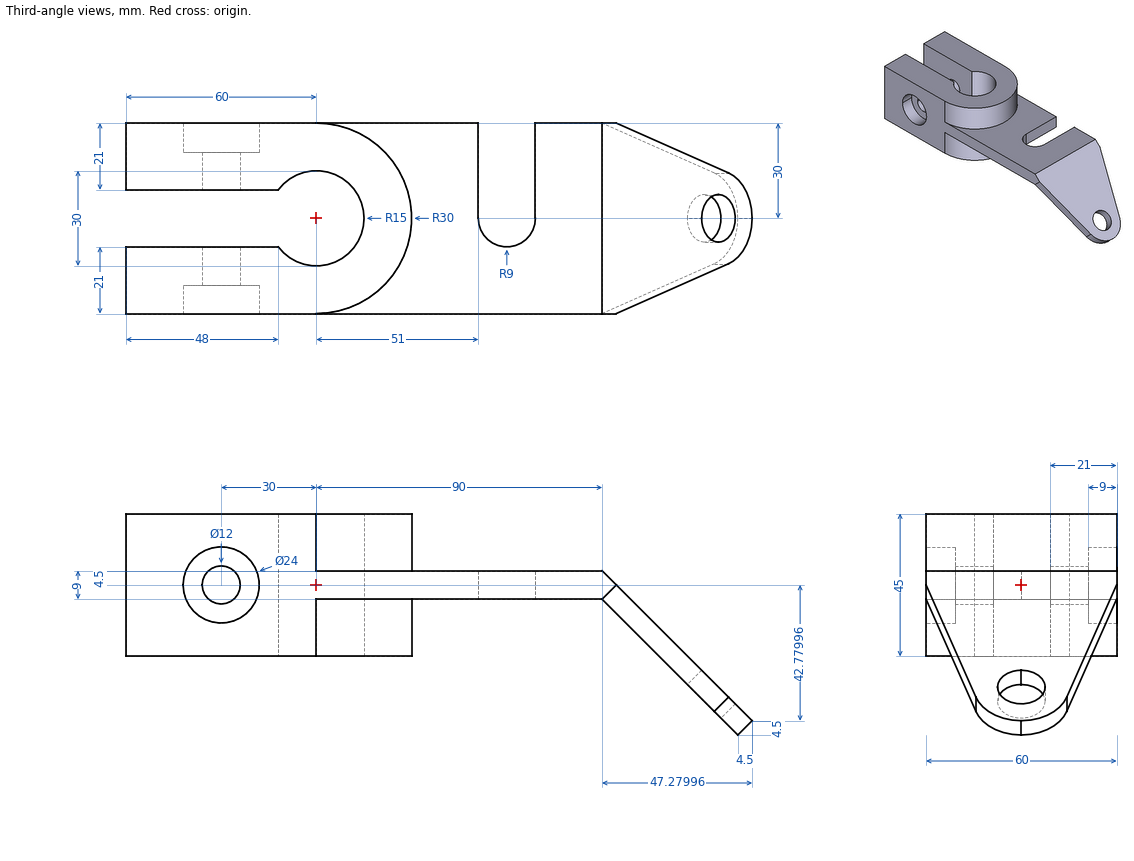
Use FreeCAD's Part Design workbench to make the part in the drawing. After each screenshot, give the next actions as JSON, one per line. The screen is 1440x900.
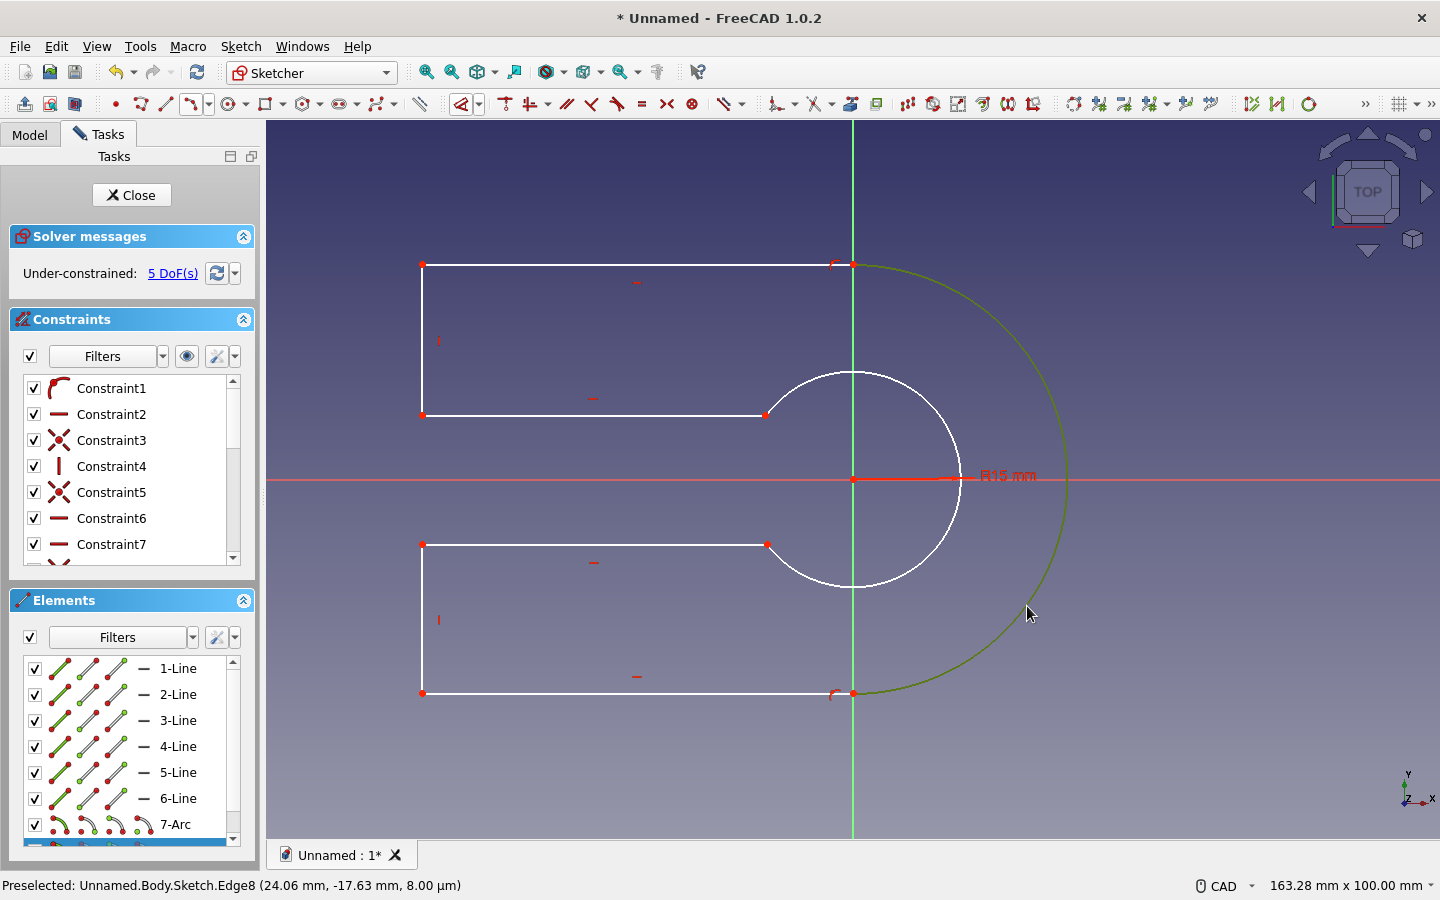
{"action": "left_click", "coordinate": [478, 104]}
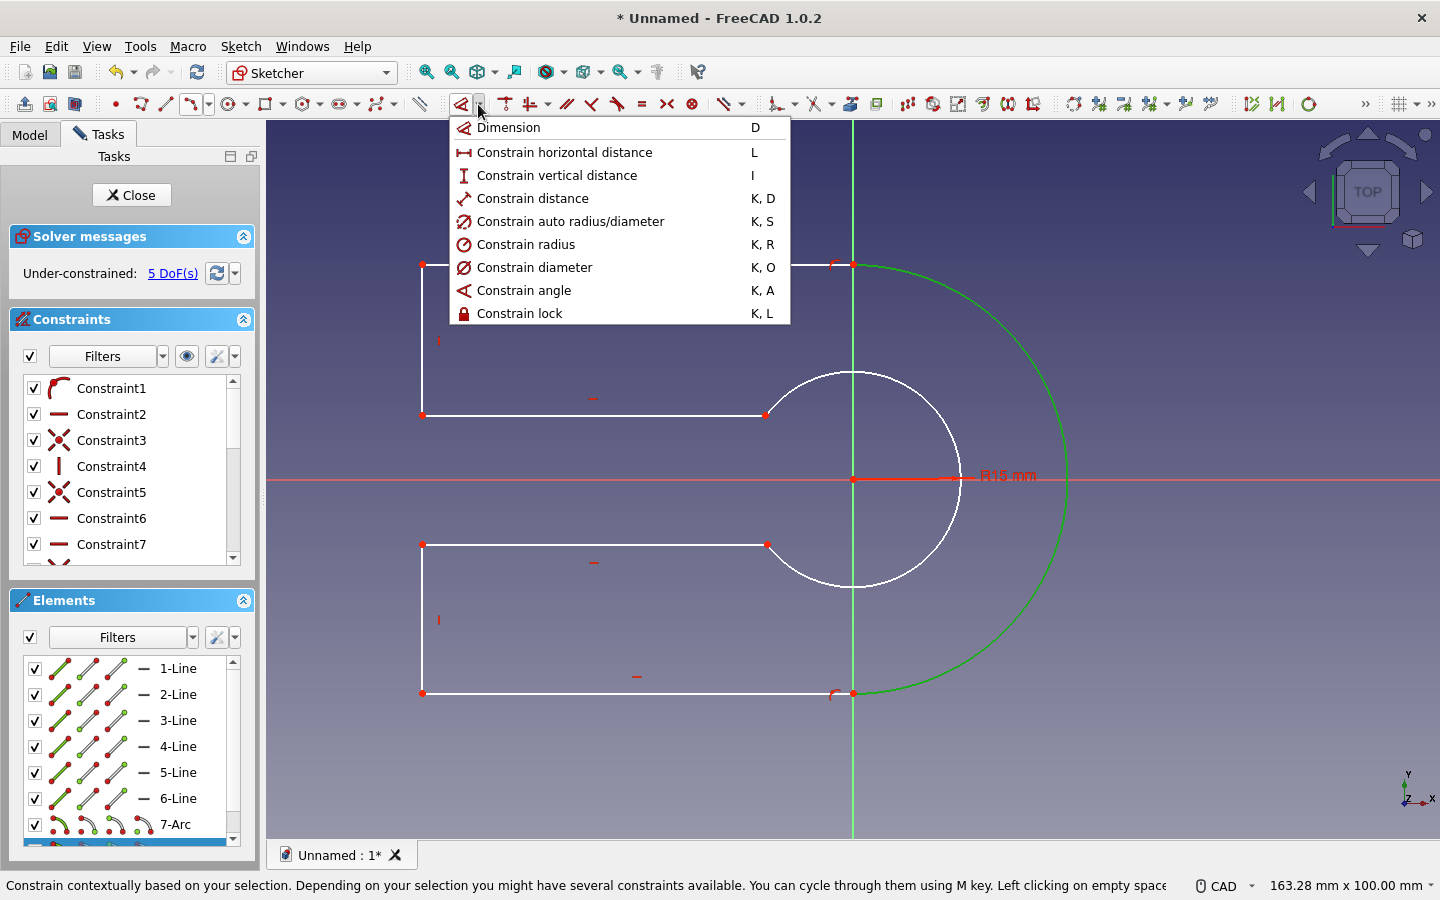
{"action": "left_click", "coordinate": [620, 244]}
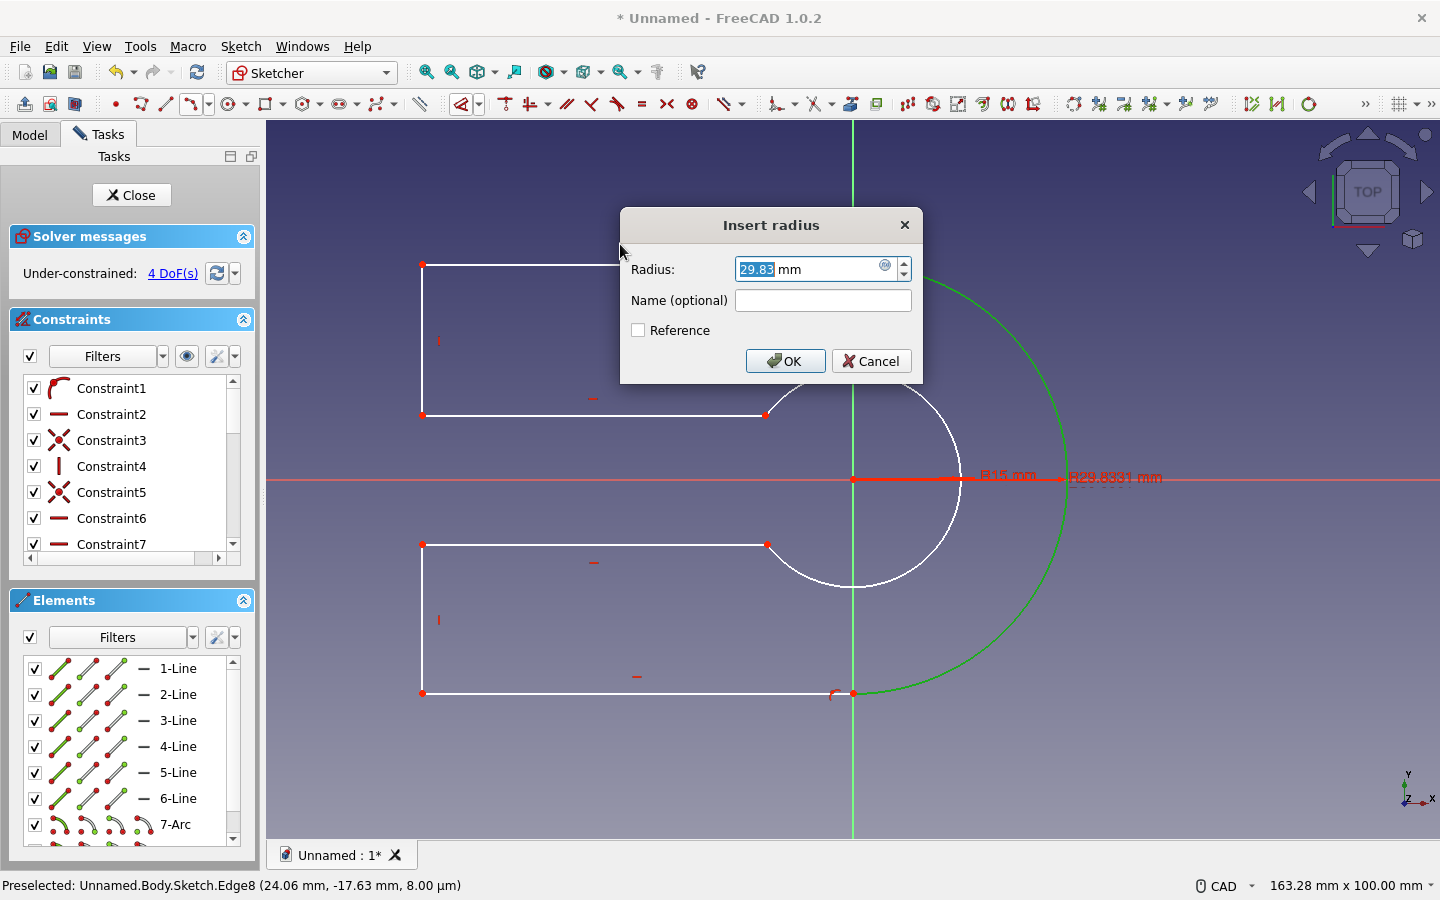
{"action": "type", "text": "30"}
{"action": "key", "text": "Return"}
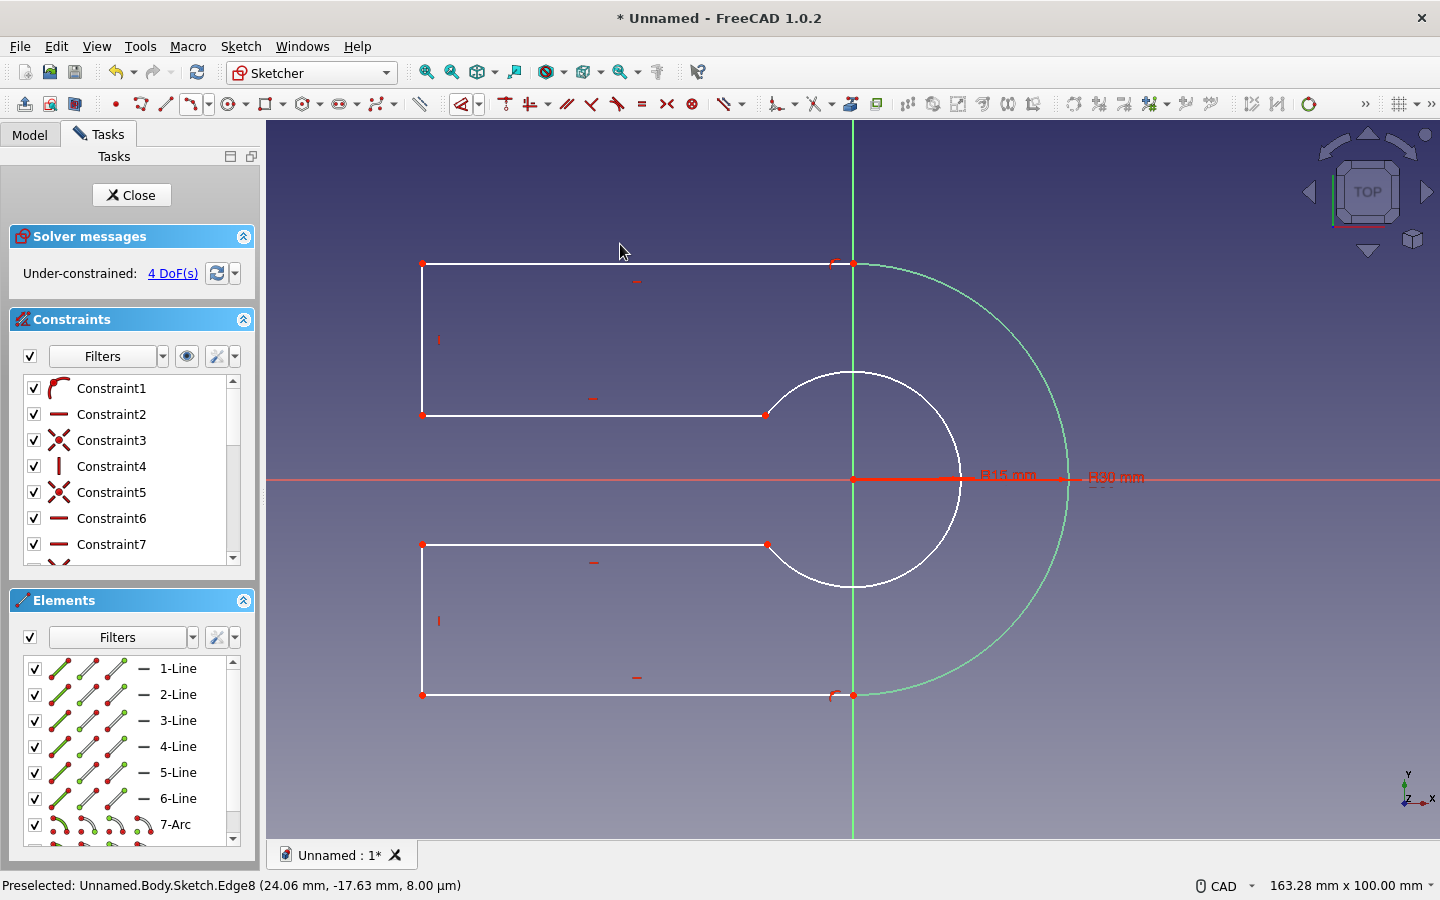
{"action": "left_click", "coordinate": [724, 264]}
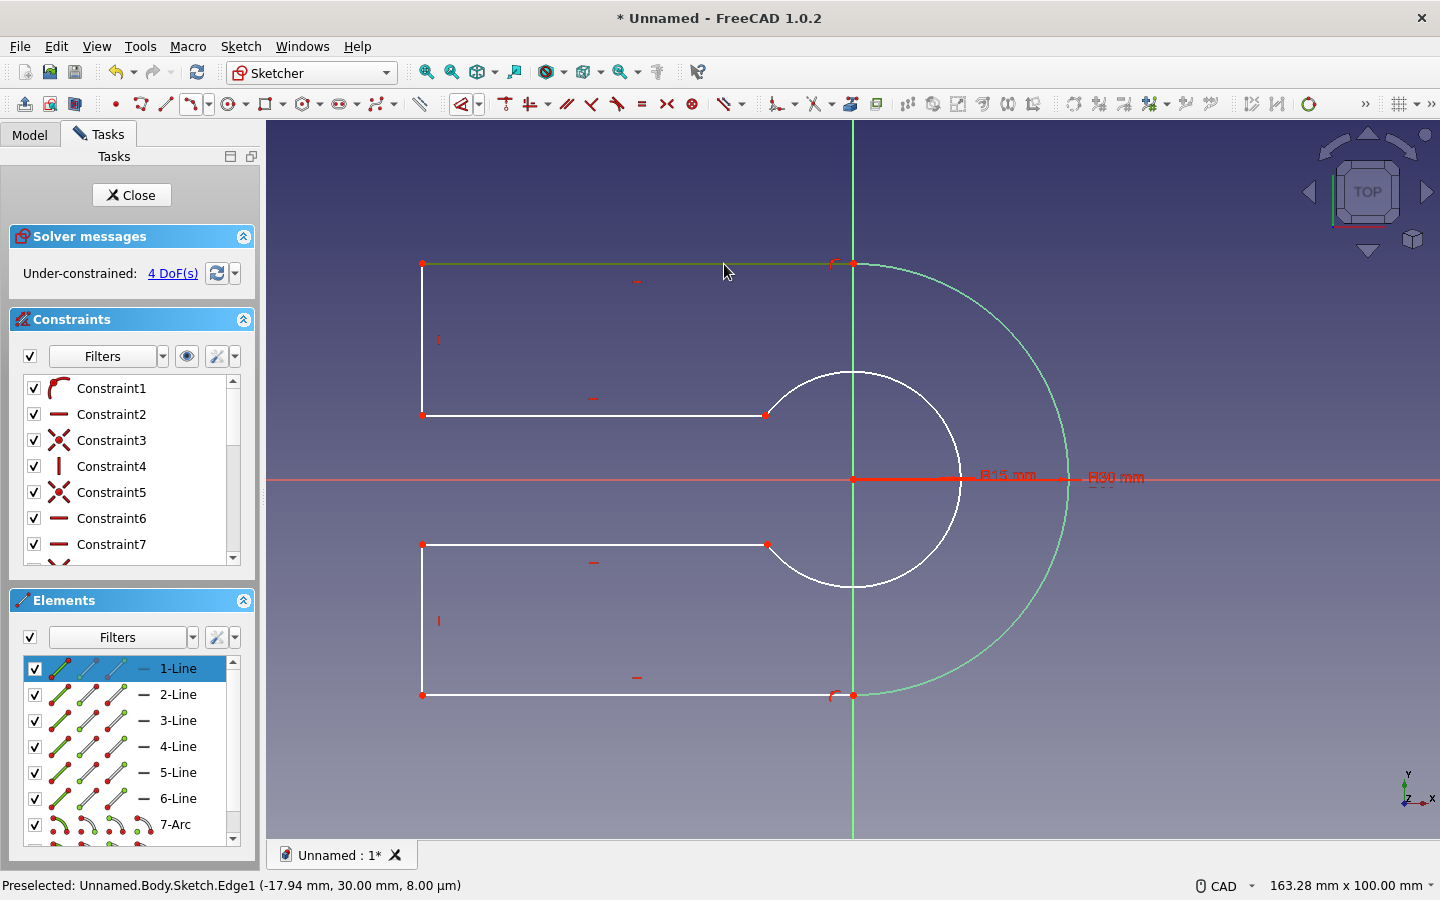
{"action": "left_click", "coordinate": [478, 104]}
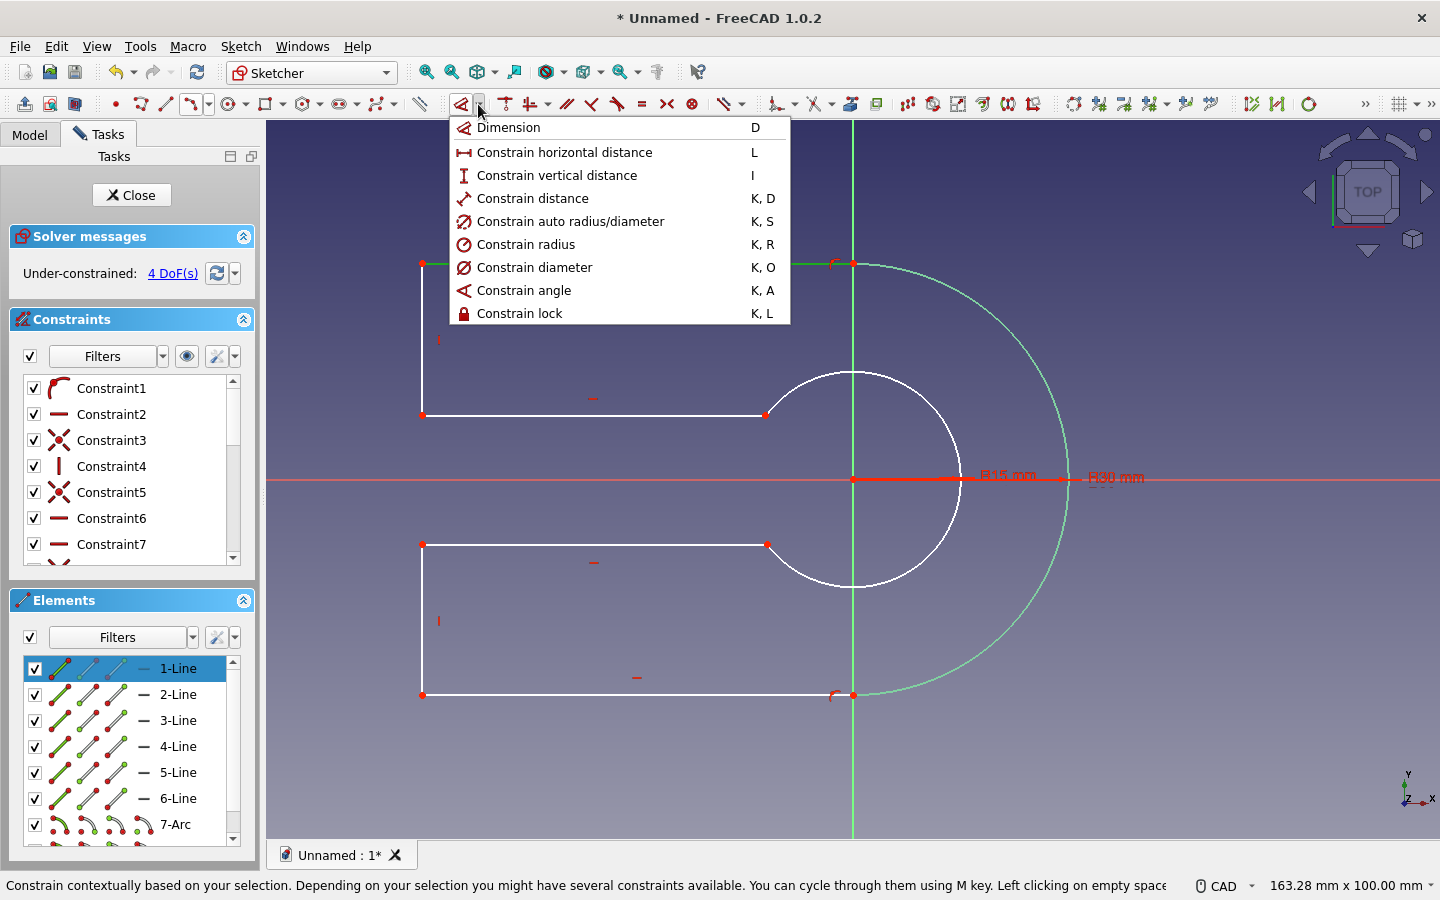
{"action": "left_click", "coordinate": [620, 152]}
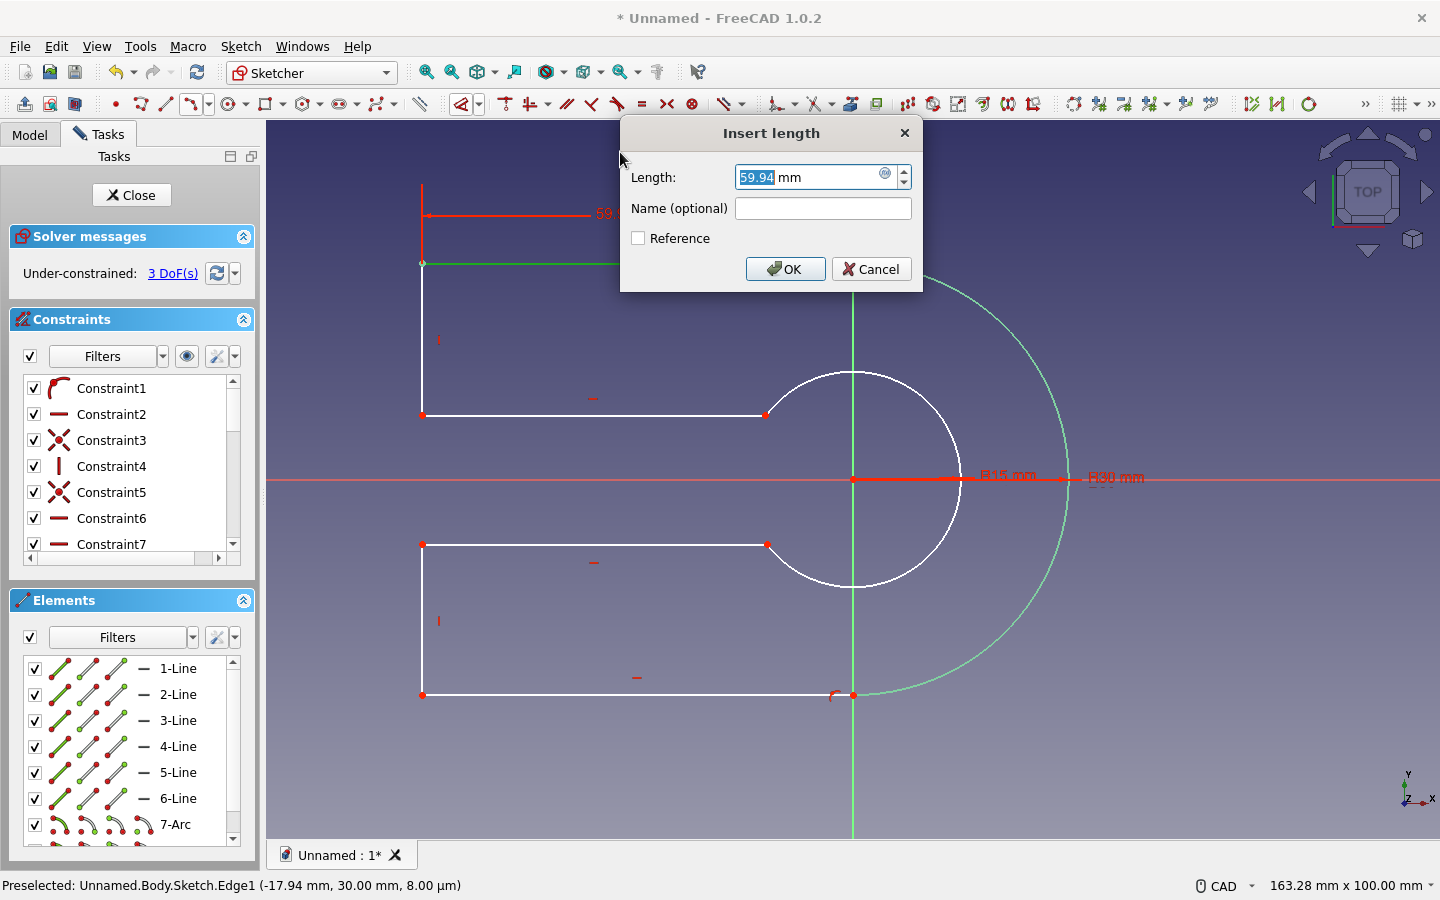
{"action": "type", "text": "60"}
{"action": "key", "text": "Return"}